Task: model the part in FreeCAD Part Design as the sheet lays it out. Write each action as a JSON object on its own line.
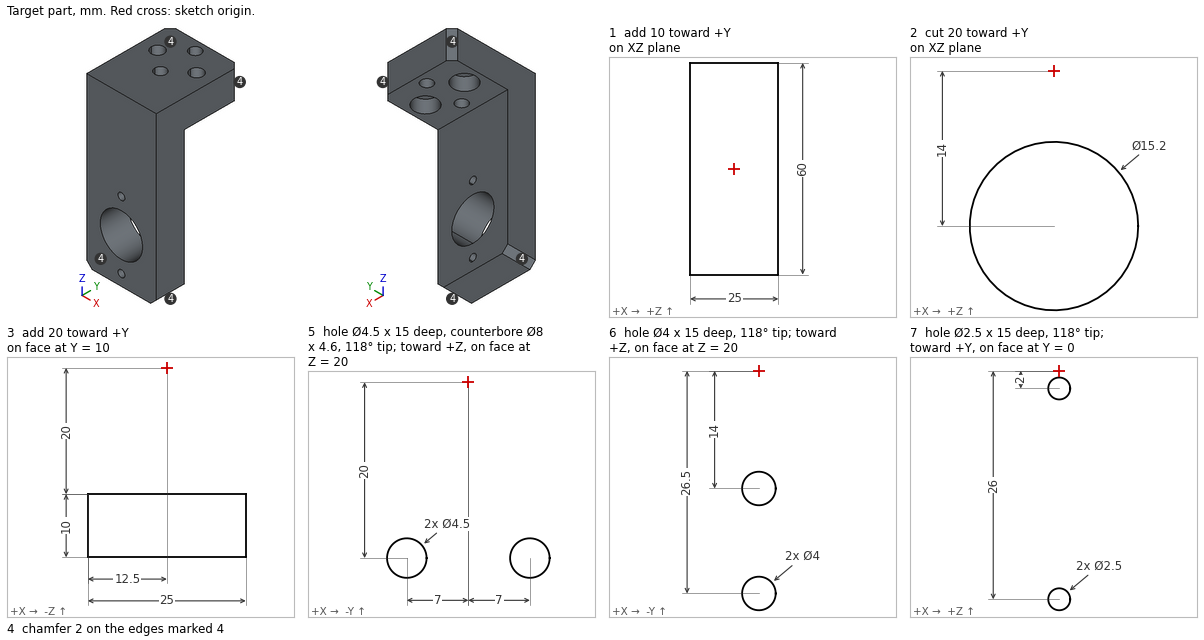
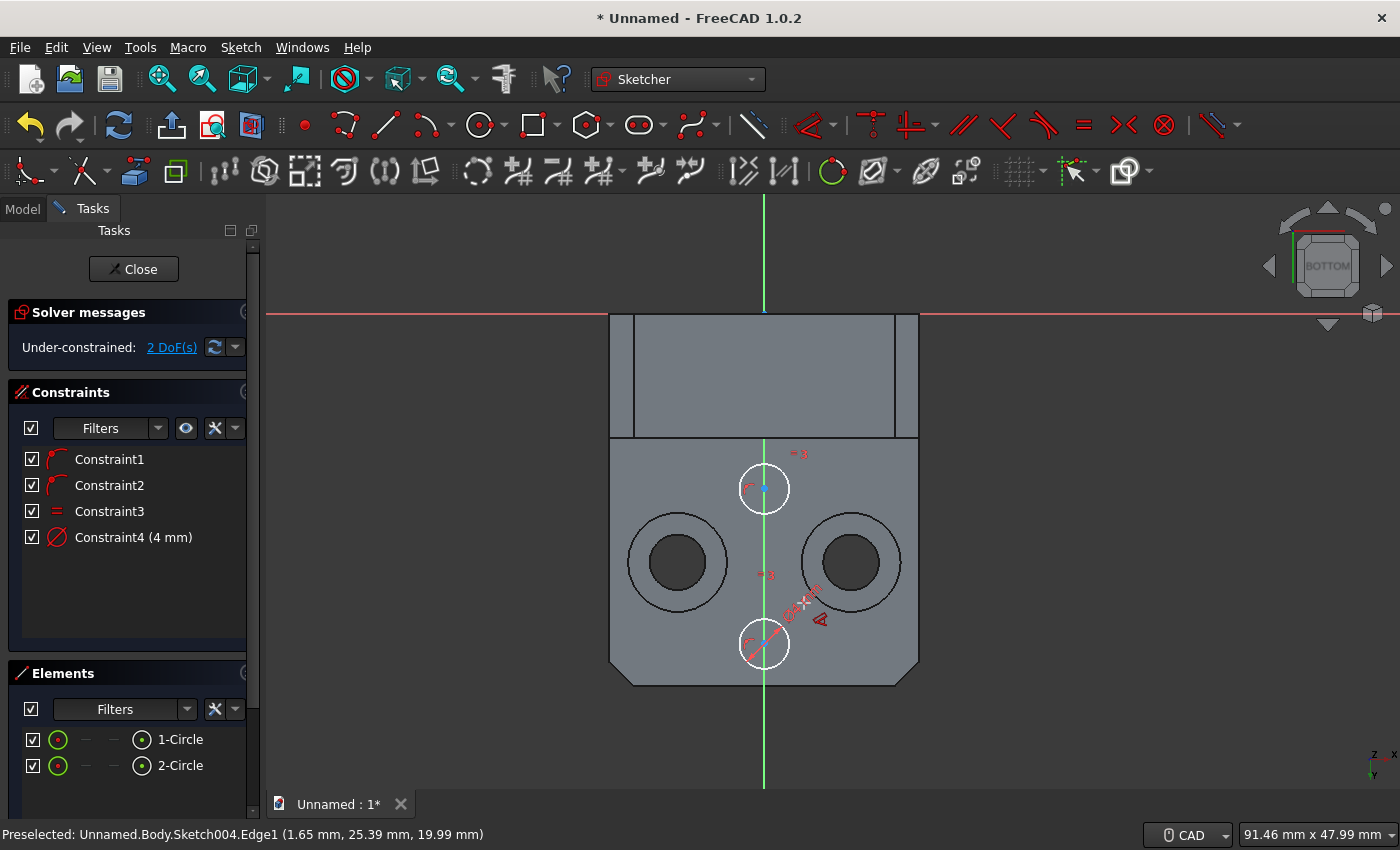
{"action": "left_click", "coordinate": [764, 489]}
{"action": "left_click", "coordinate": [798, 402]}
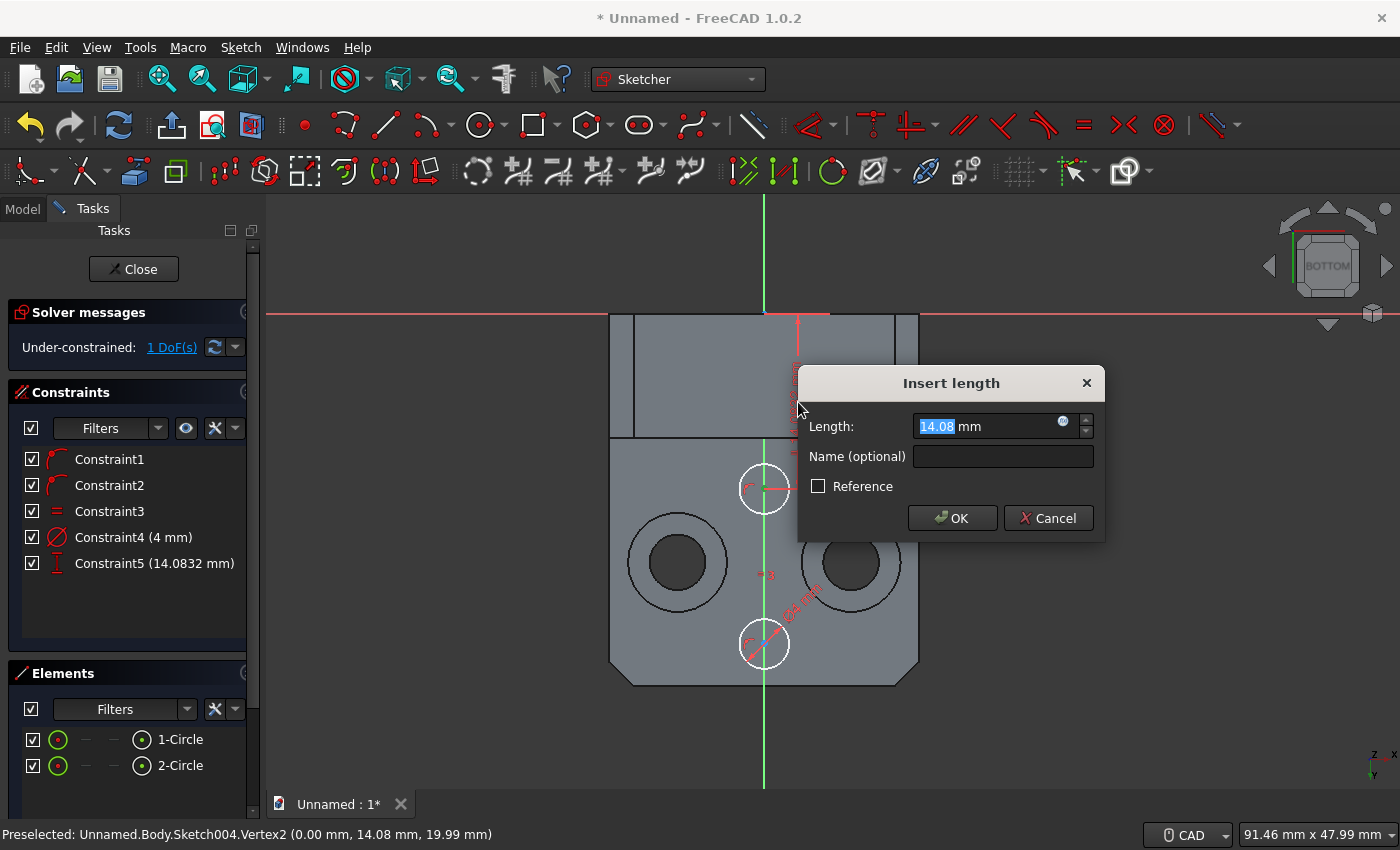
{"action": "type", "text": "14"}
{"action": "key", "text": "Return"}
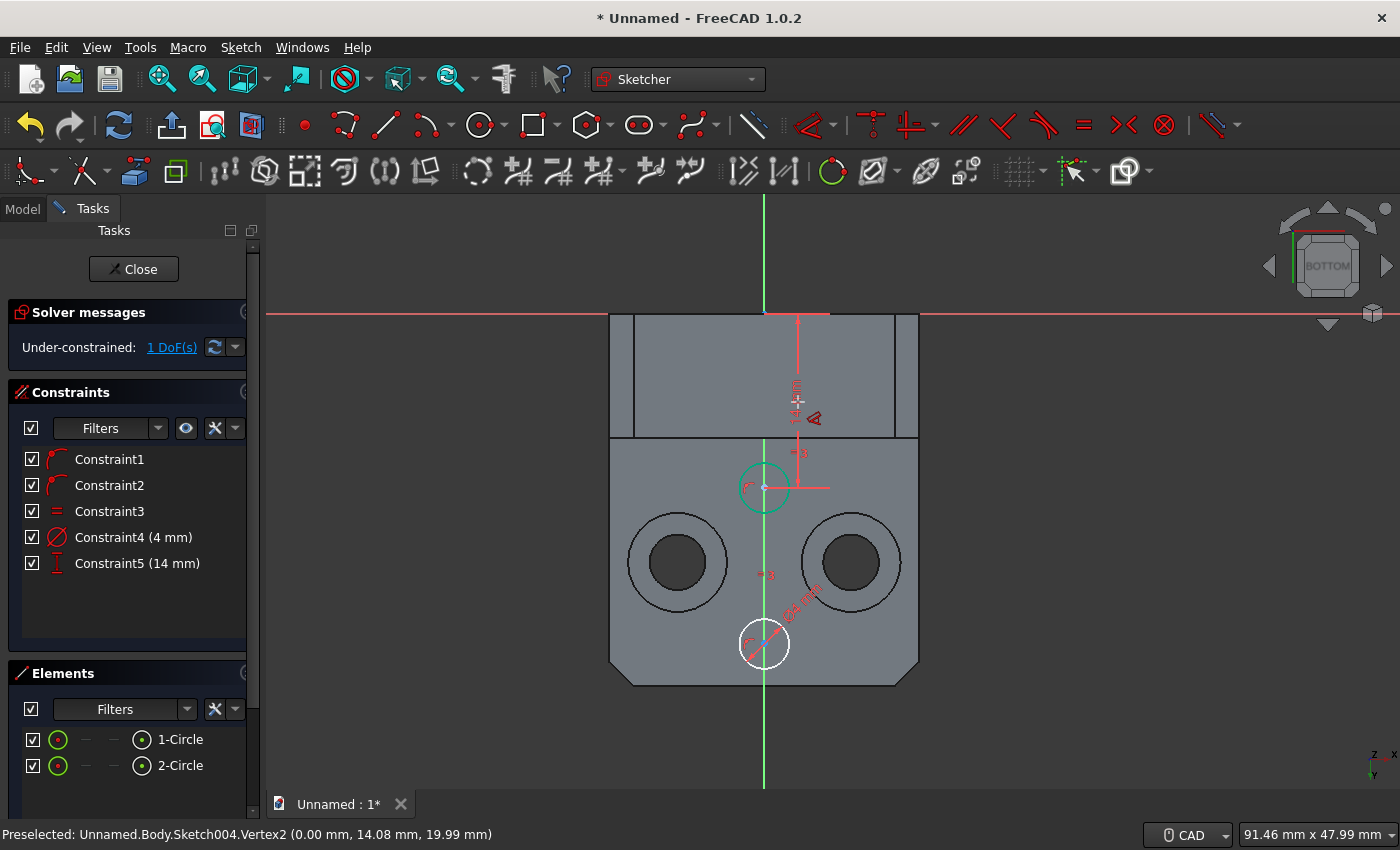
{"action": "left_click", "coordinate": [764, 644]}
{"action": "left_click", "coordinate": [798, 555]}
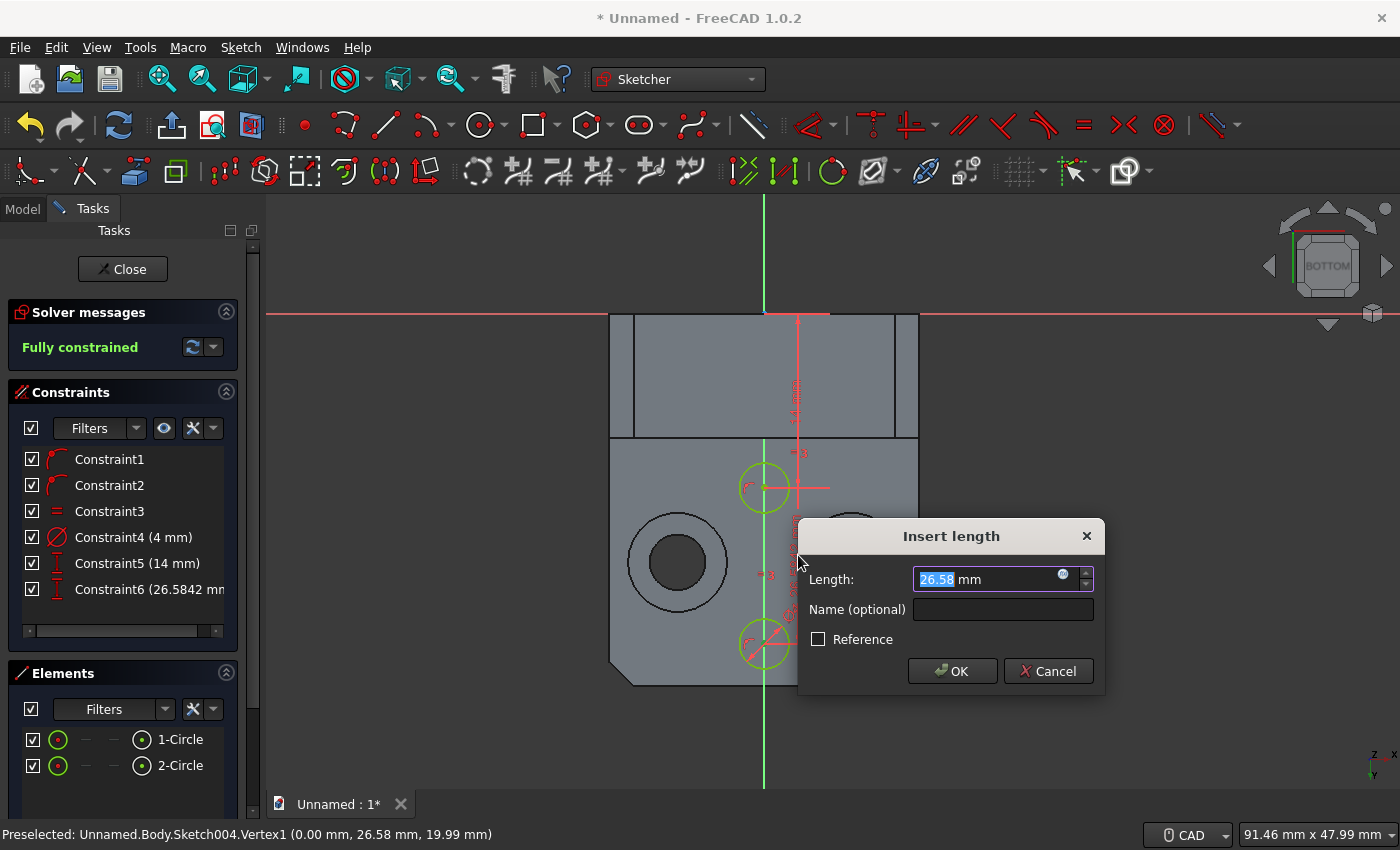
{"action": "type", "text": "26.5"}
{"action": "key", "text": "Return"}
{"action": "key", "text": "Escape"}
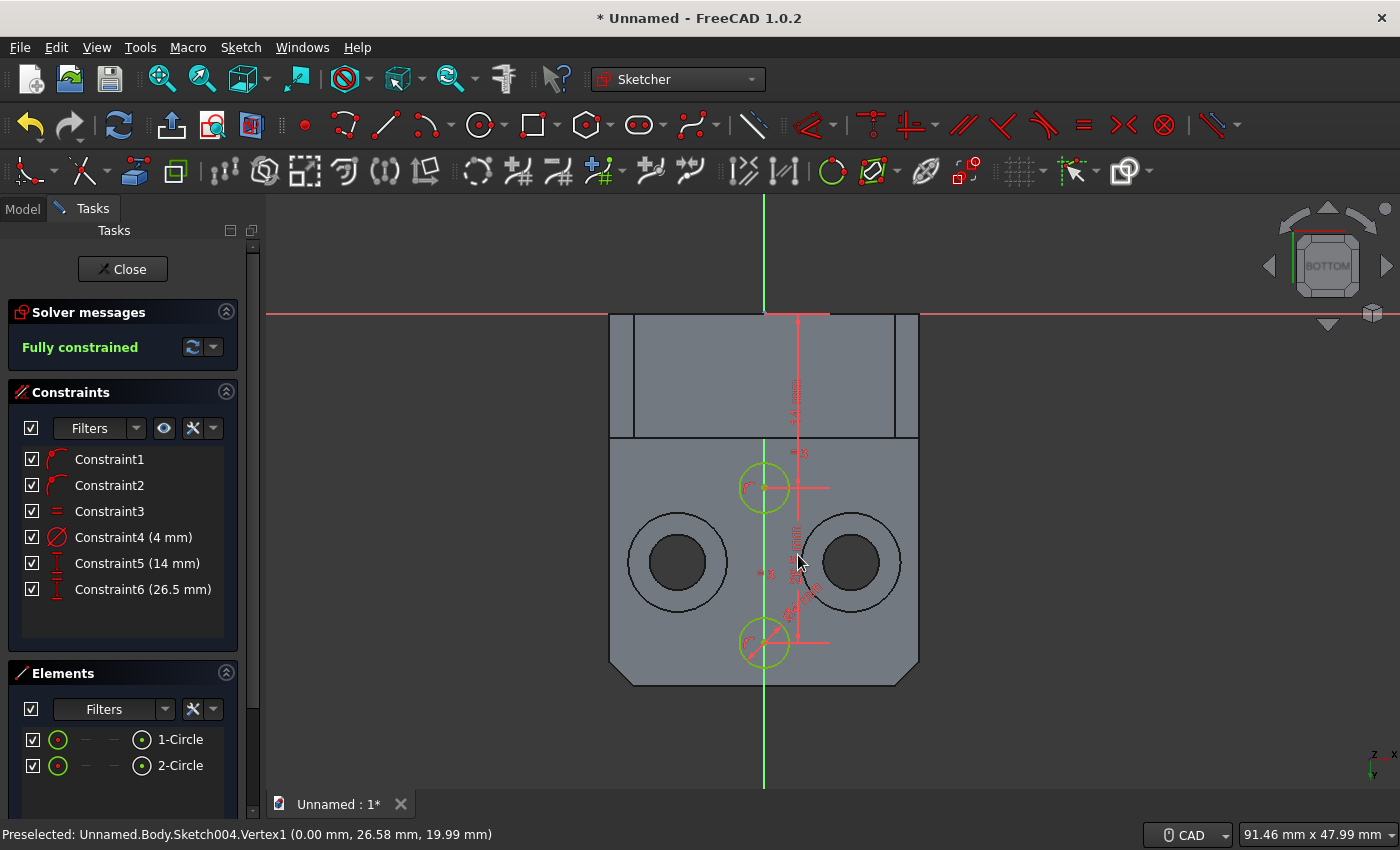
{"action": "left_click", "coordinate": [123, 269]}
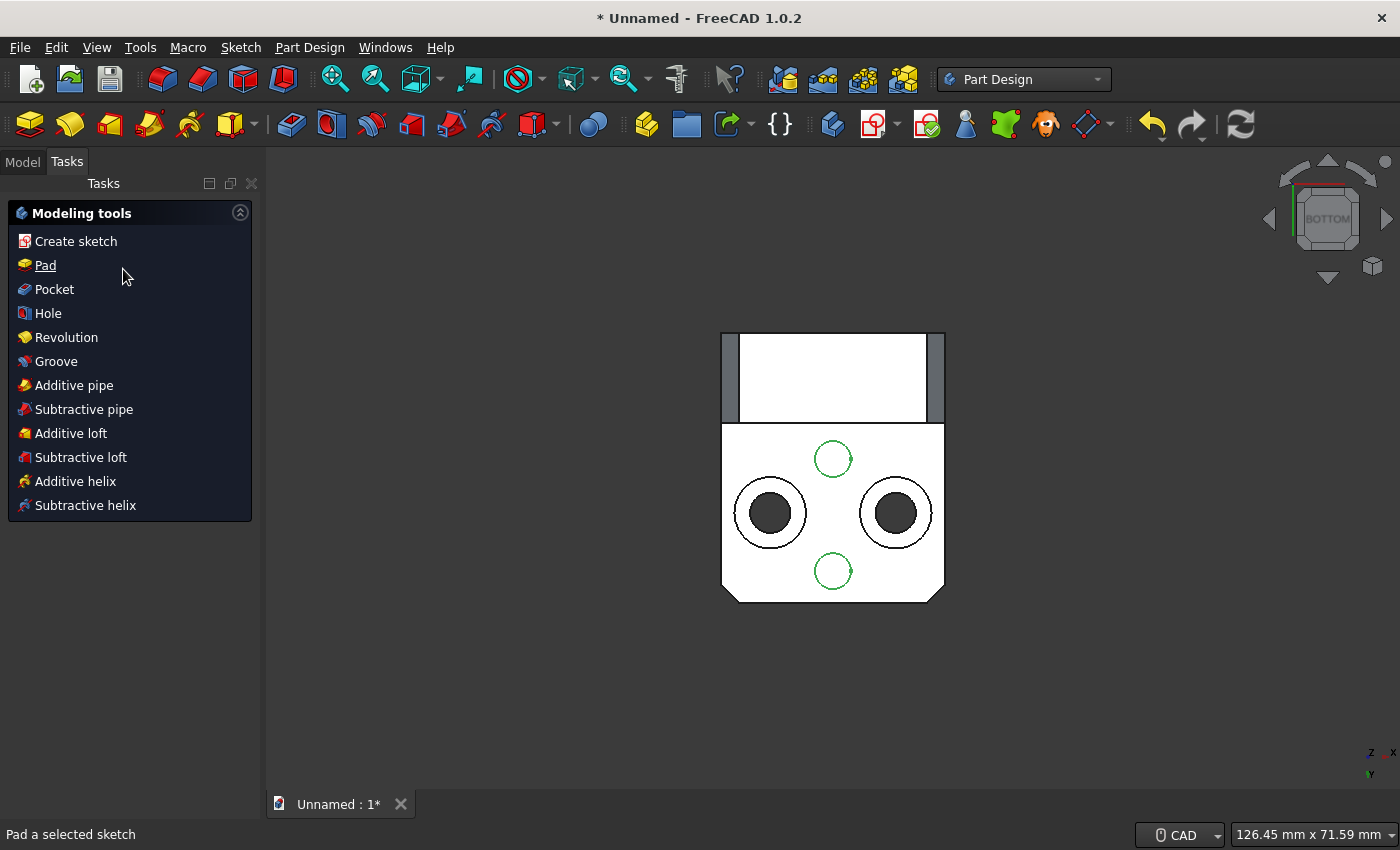
{"action": "left_click", "coordinate": [332, 124]}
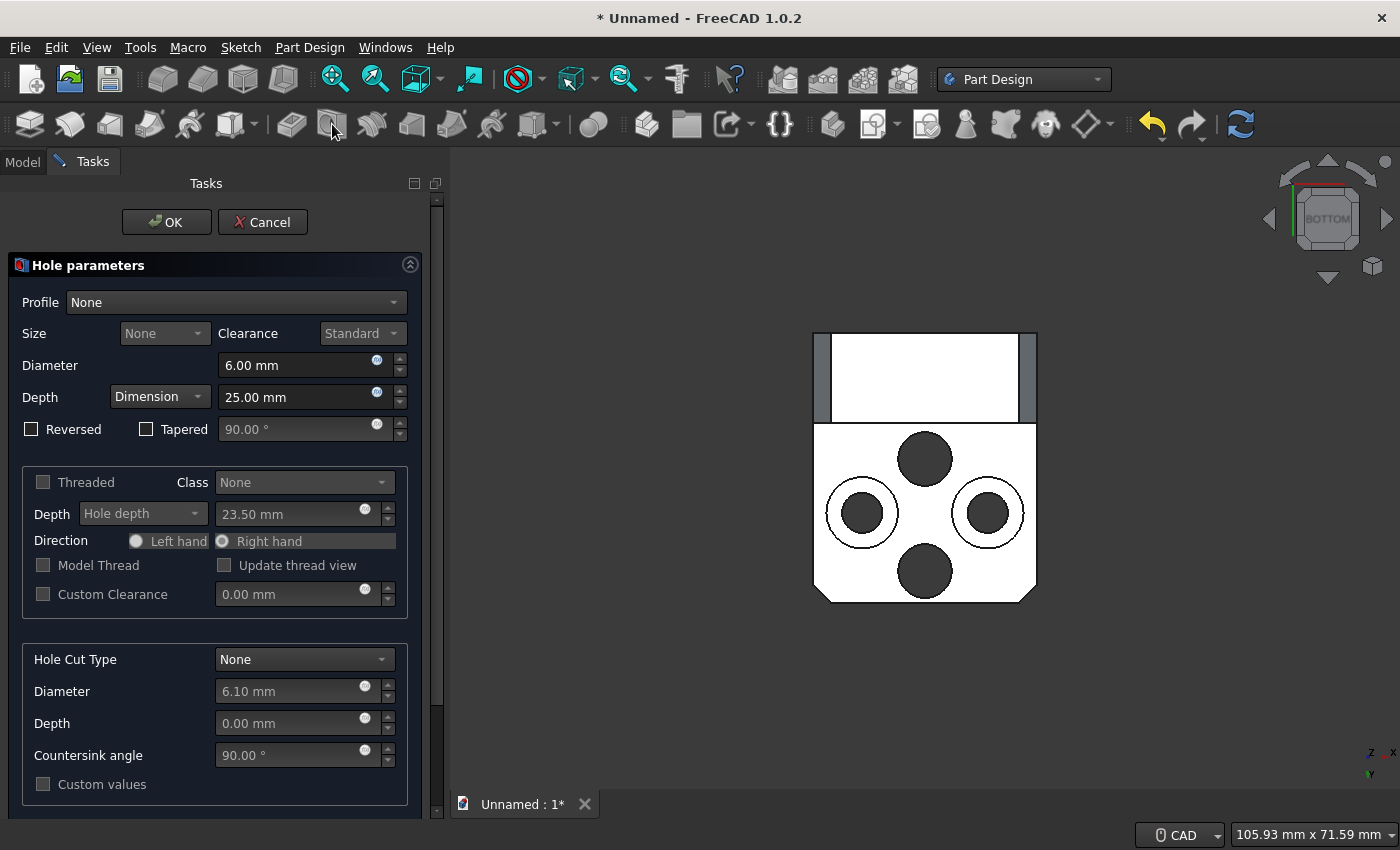
{"action": "triple_click", "coordinate": [305, 365]}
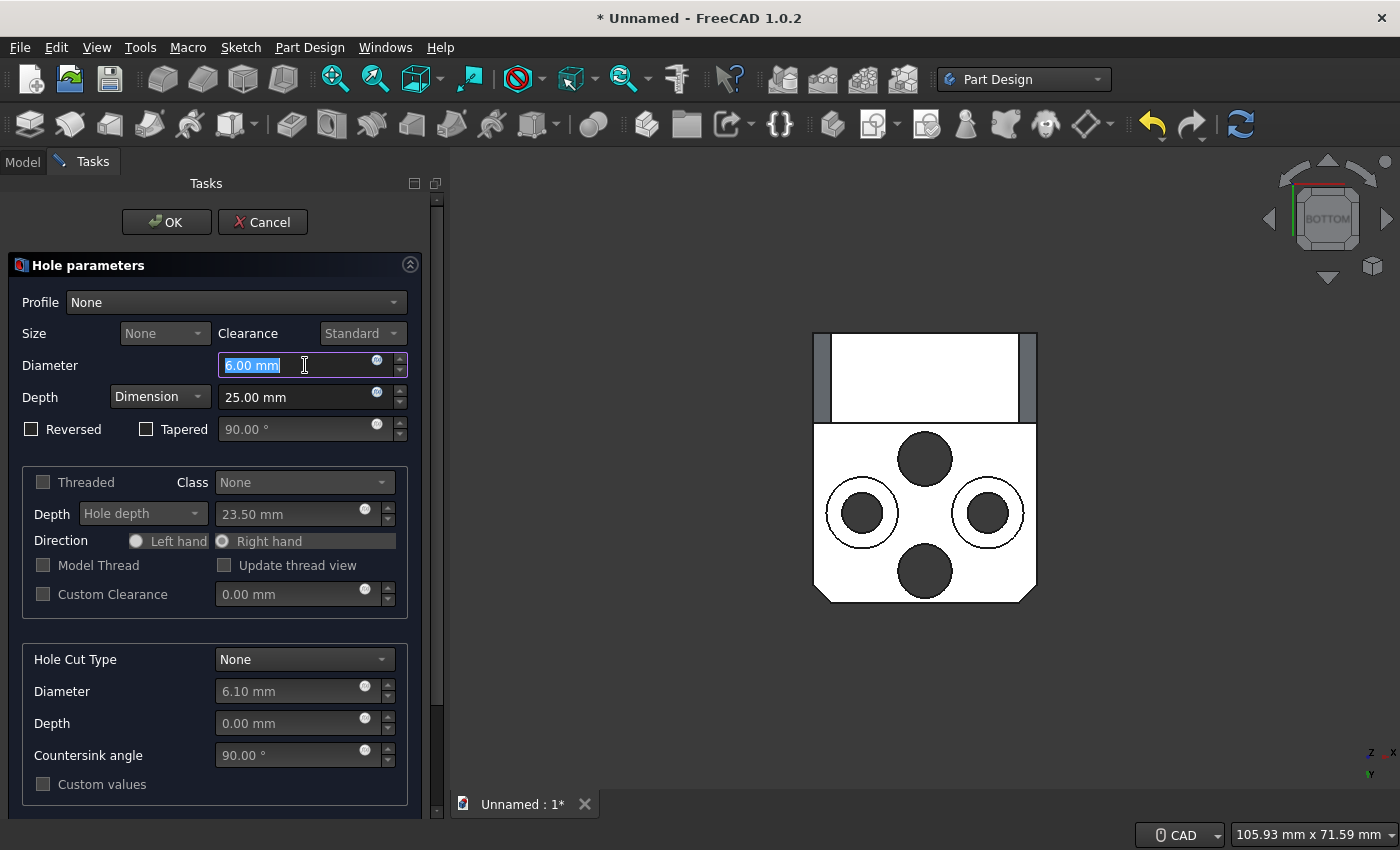
{"action": "type", "text": "4"}
{"action": "key", "text": "Tab"}